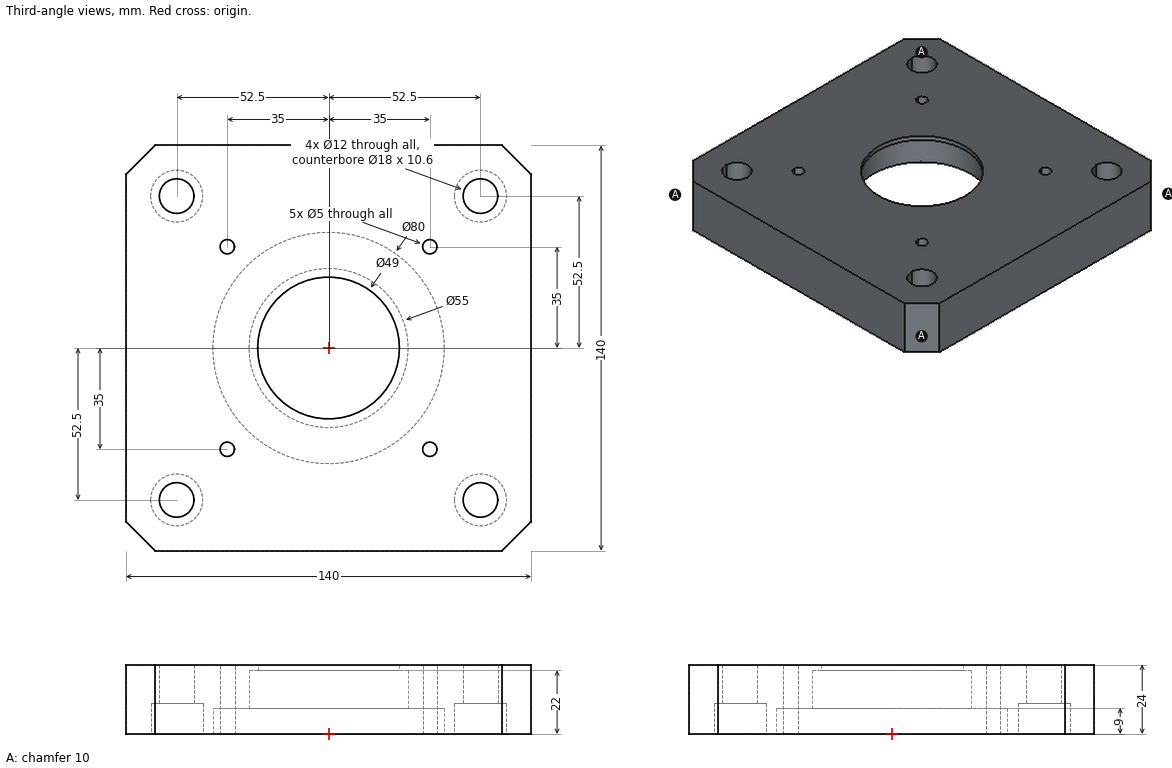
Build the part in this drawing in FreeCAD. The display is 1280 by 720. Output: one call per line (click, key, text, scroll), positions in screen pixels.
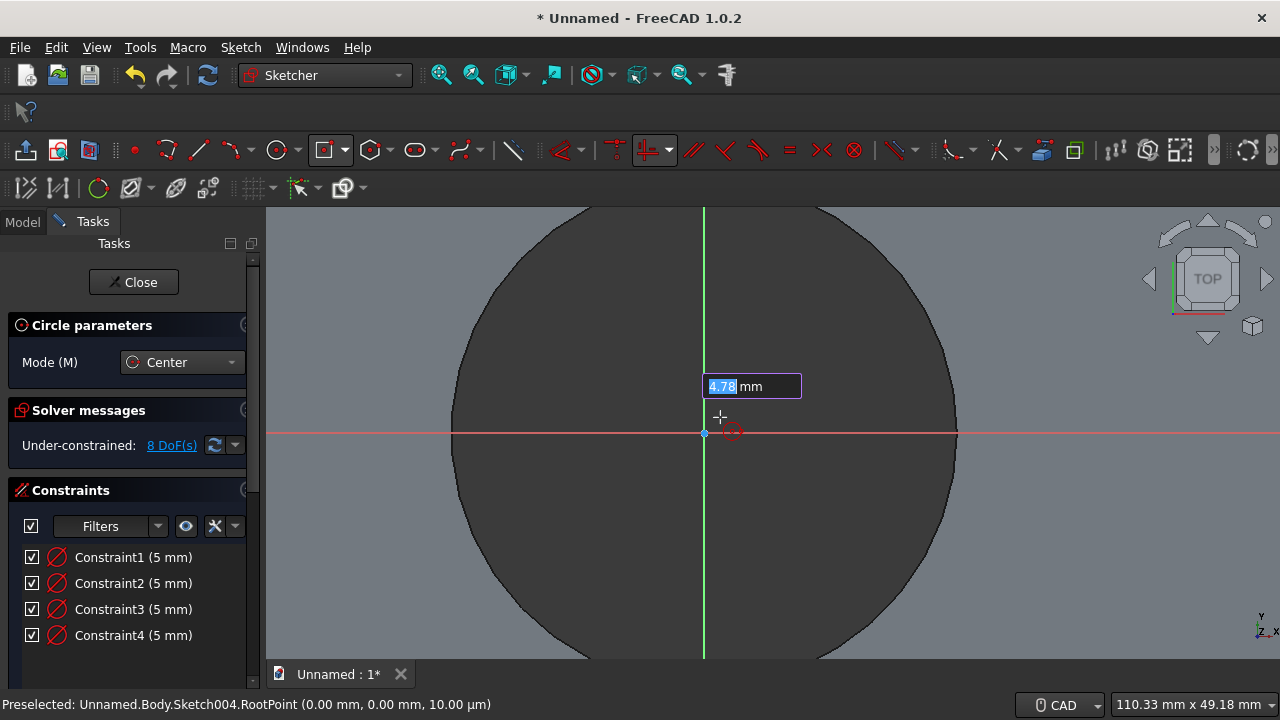
text(5)
key(Return)
key(Escape)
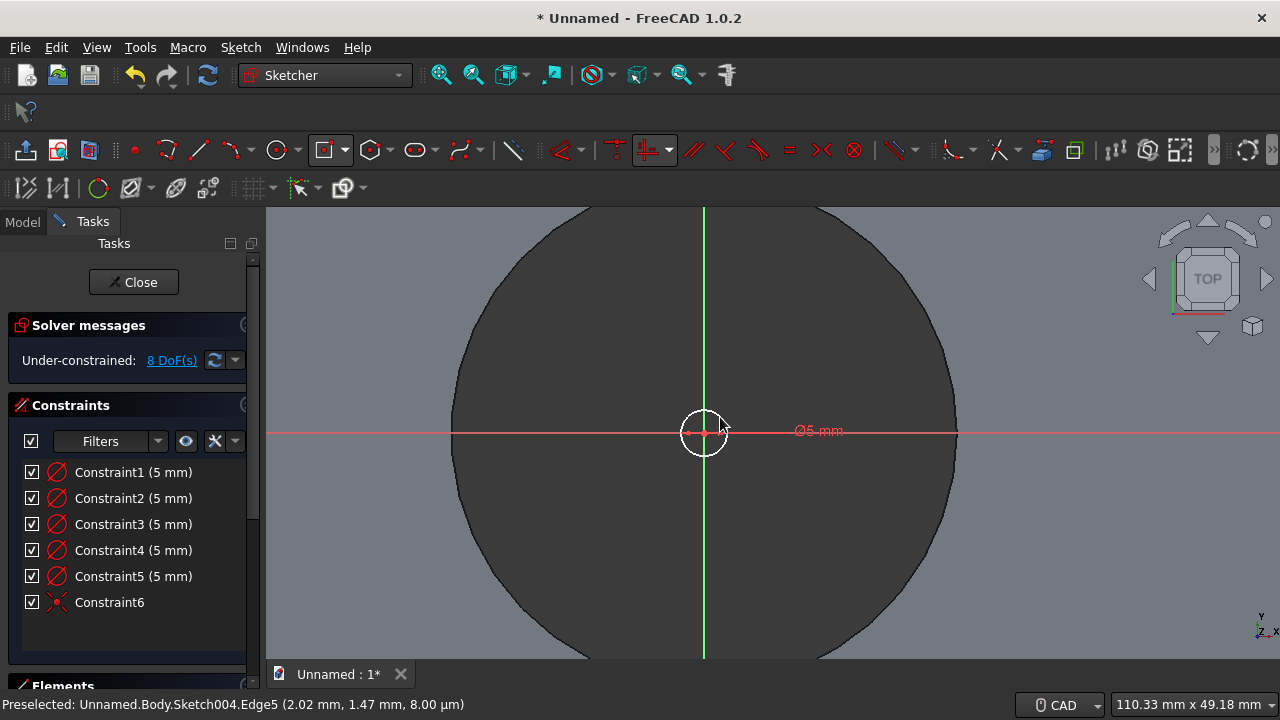
scroll(705, 433, down, 5)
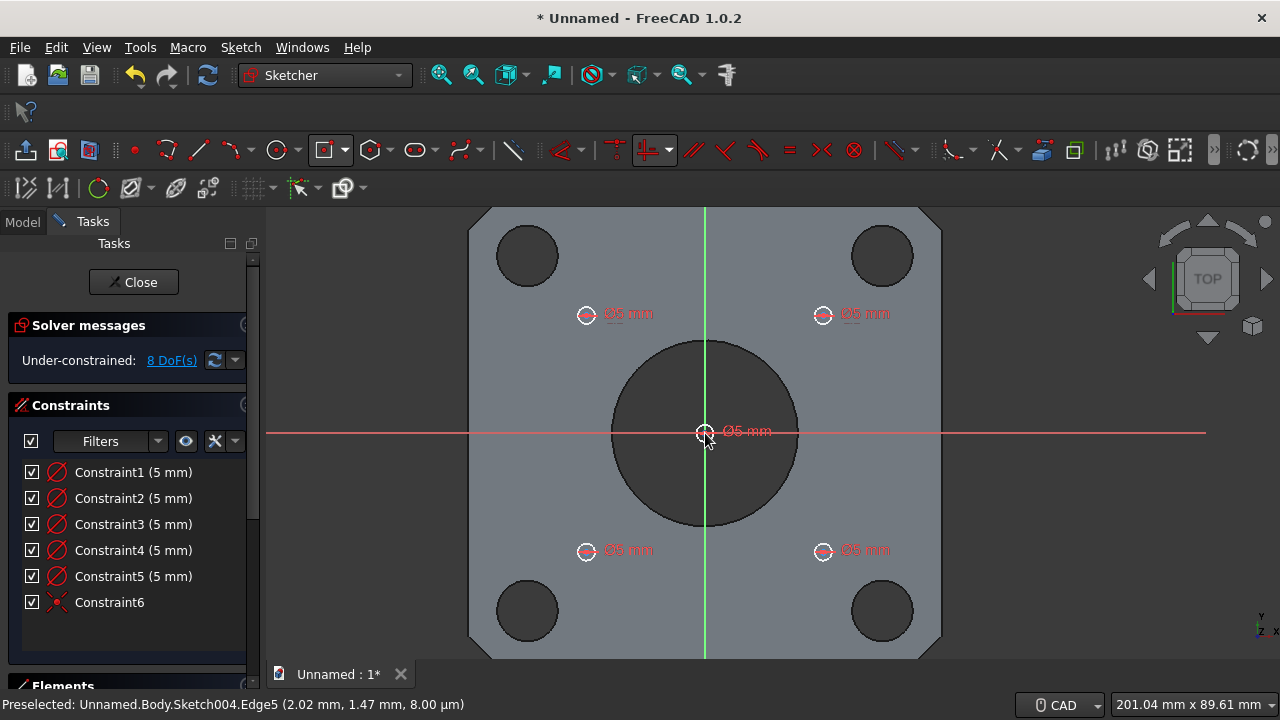
click(823, 316)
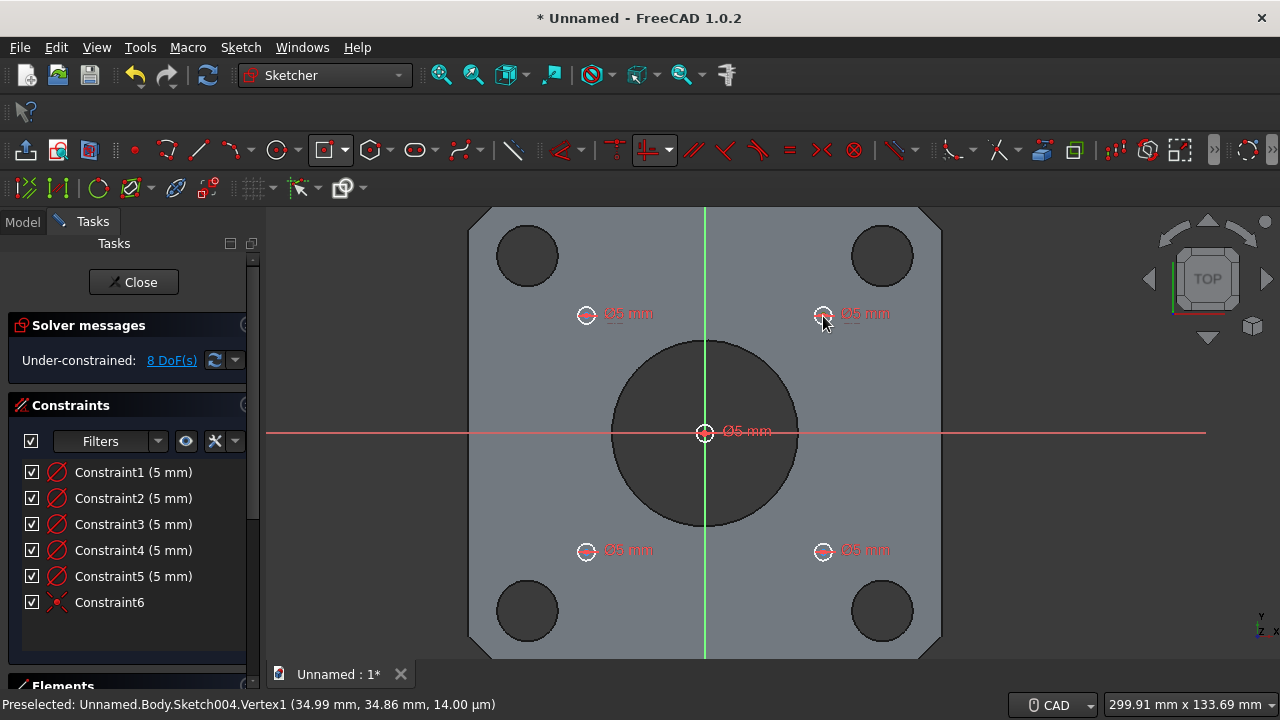
click(586, 316)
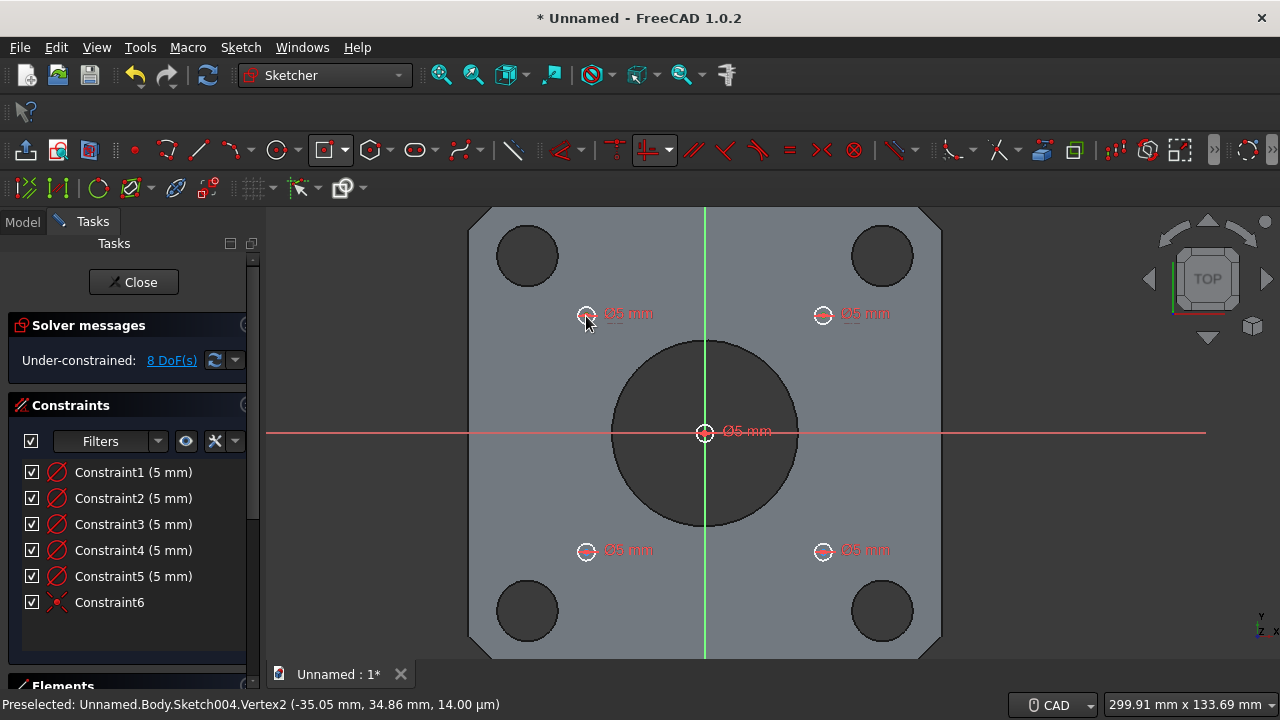
click(672, 150)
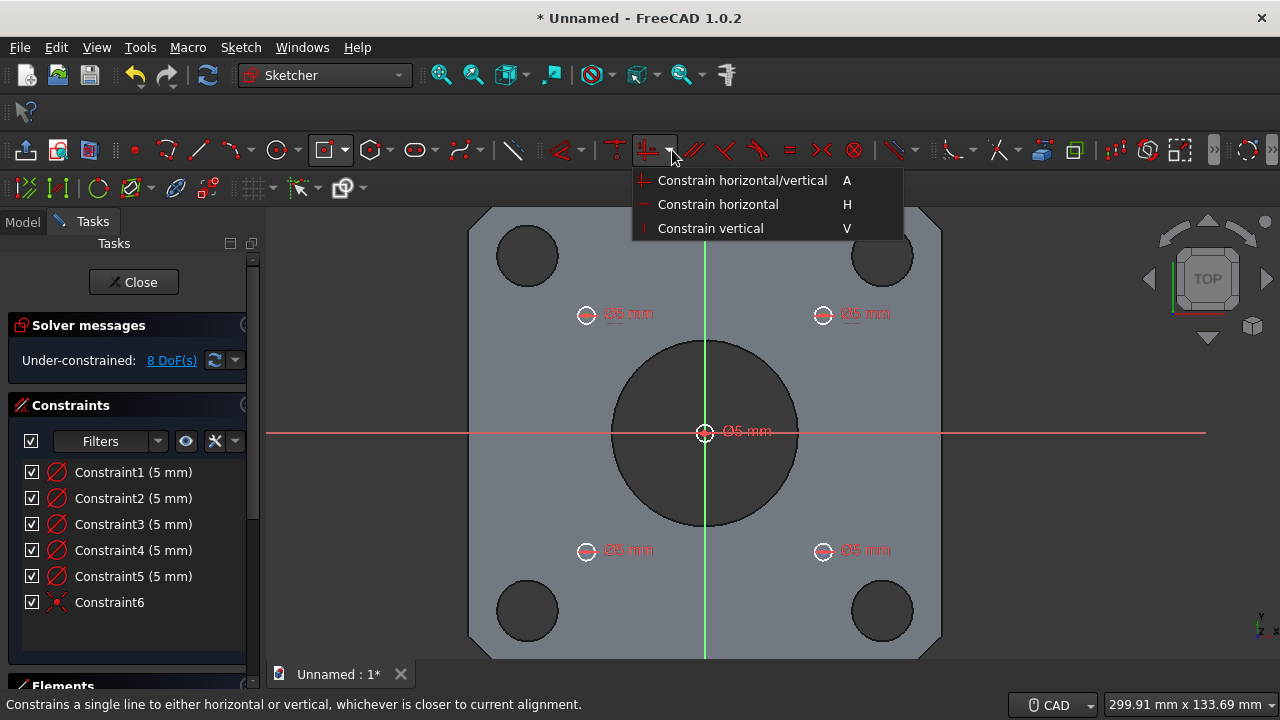
click(768, 204)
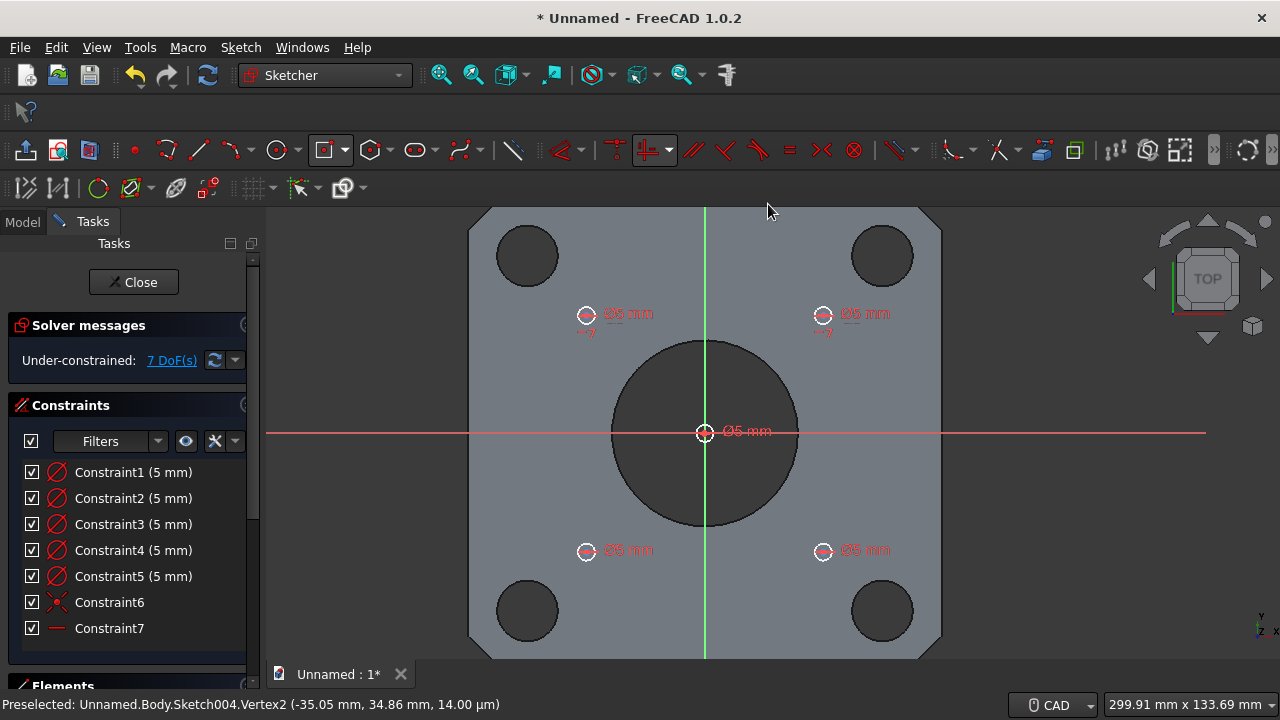
click(586, 316)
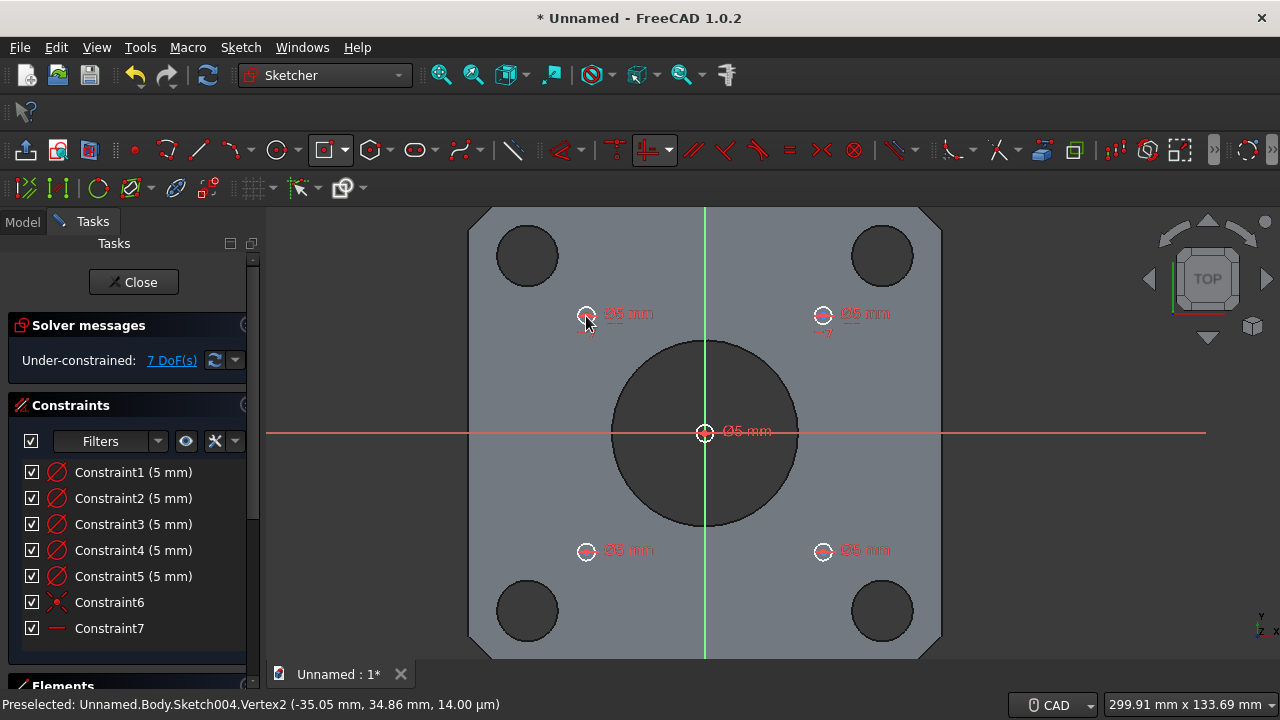
click(586, 552)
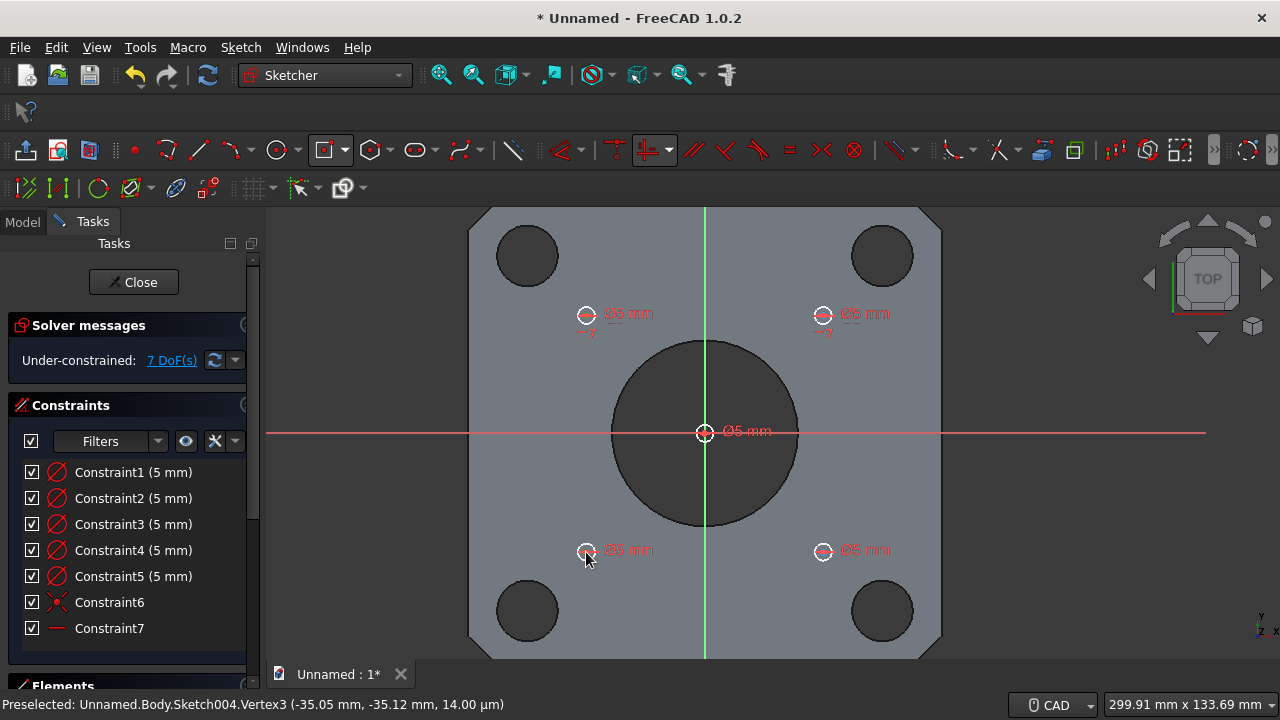
click(672, 150)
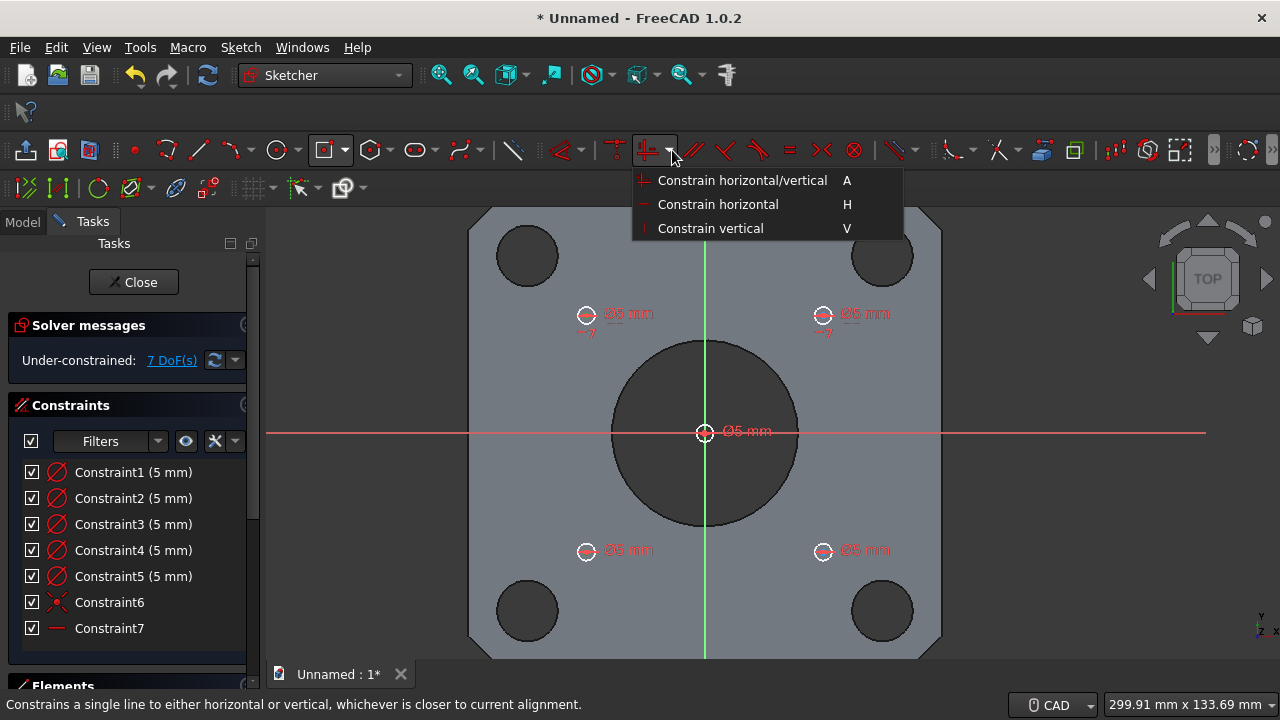
click(768, 228)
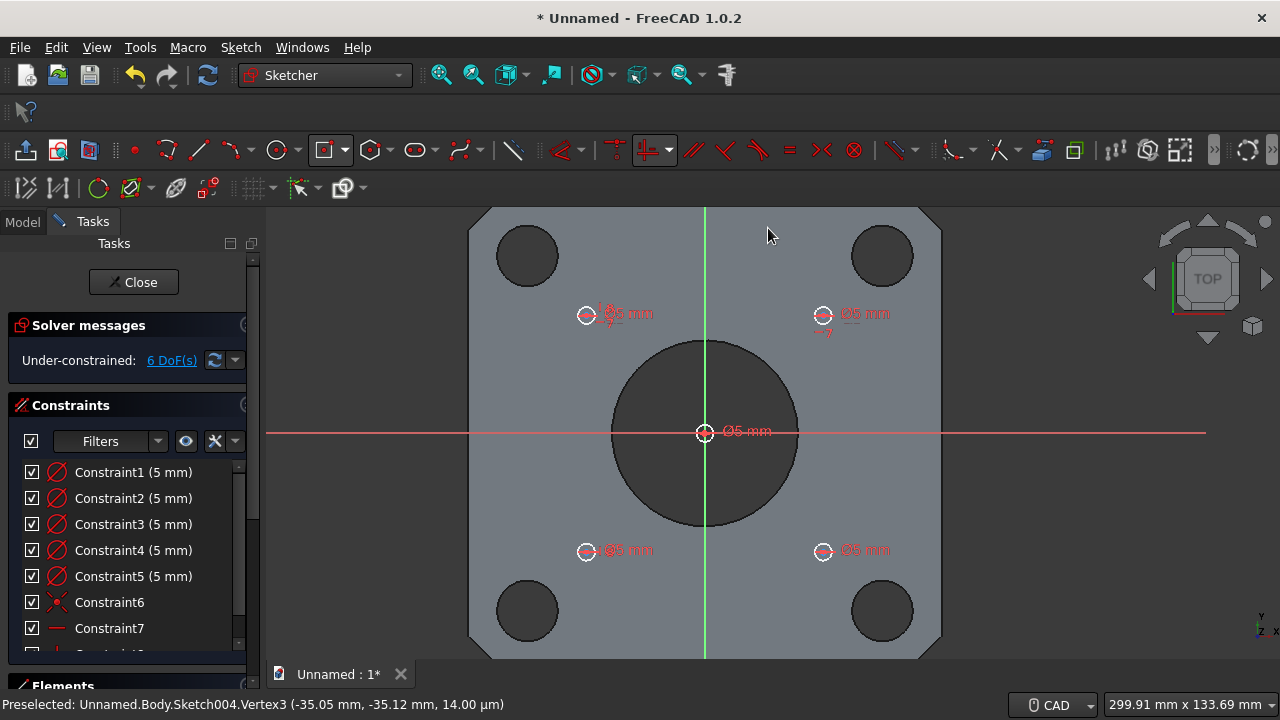
click(823, 316)